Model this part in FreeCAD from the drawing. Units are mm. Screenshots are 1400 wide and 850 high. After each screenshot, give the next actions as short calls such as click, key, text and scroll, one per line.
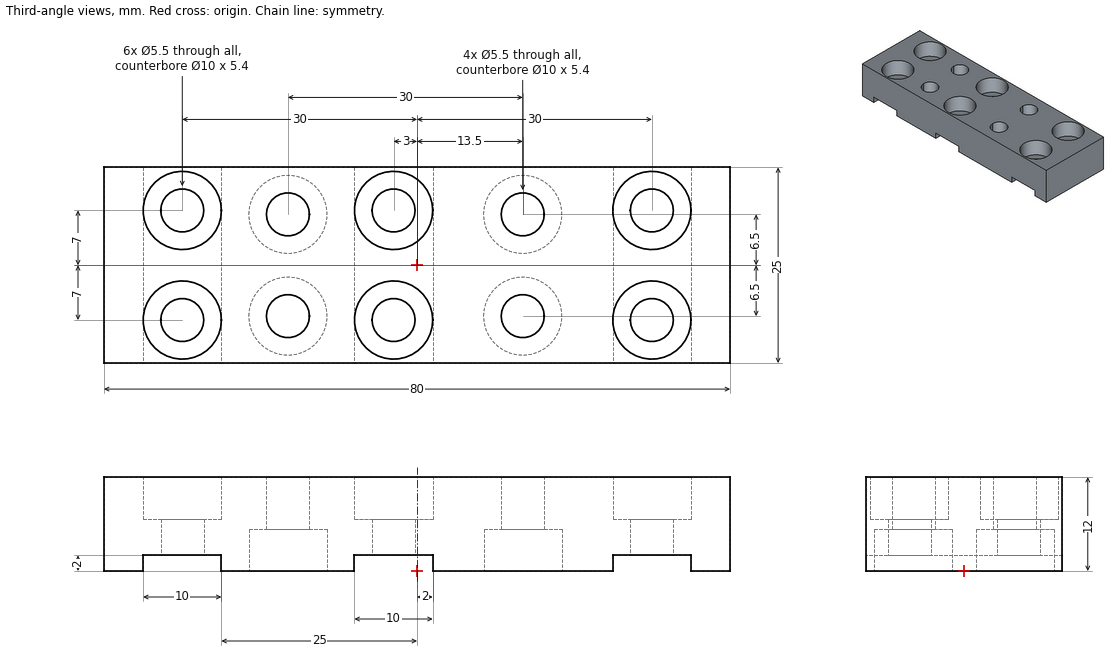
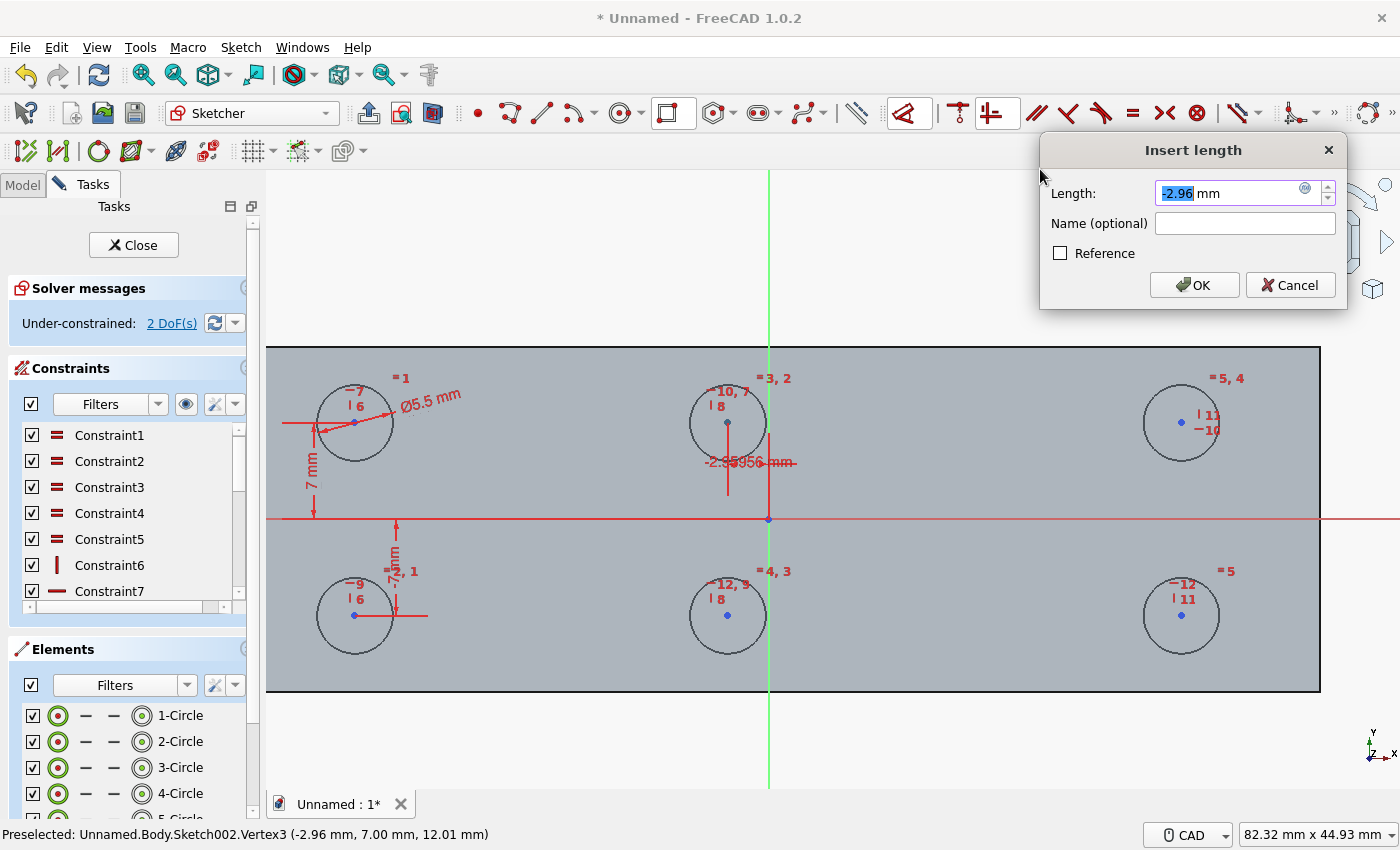
text(-3)
key(Return)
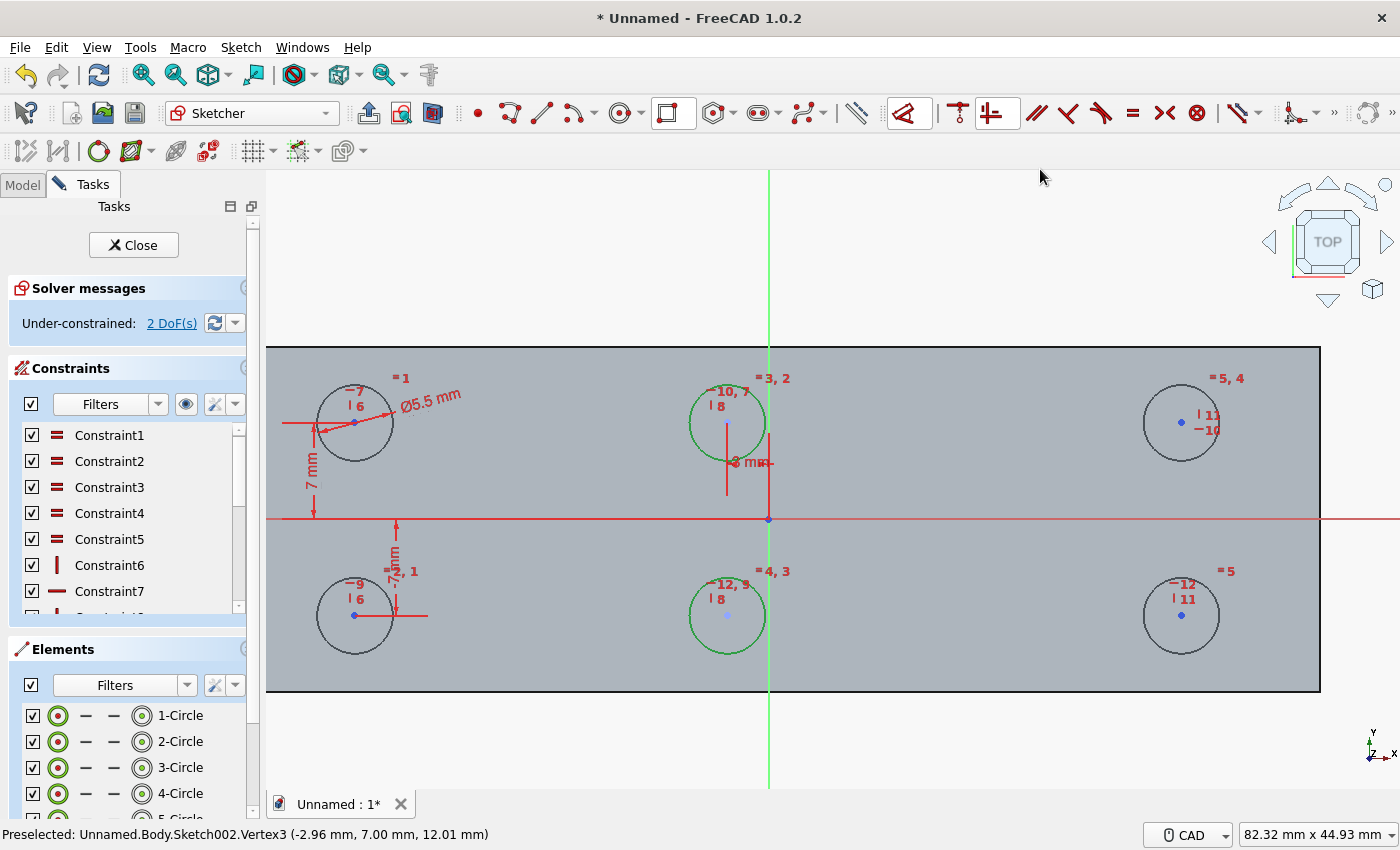
click(355, 423)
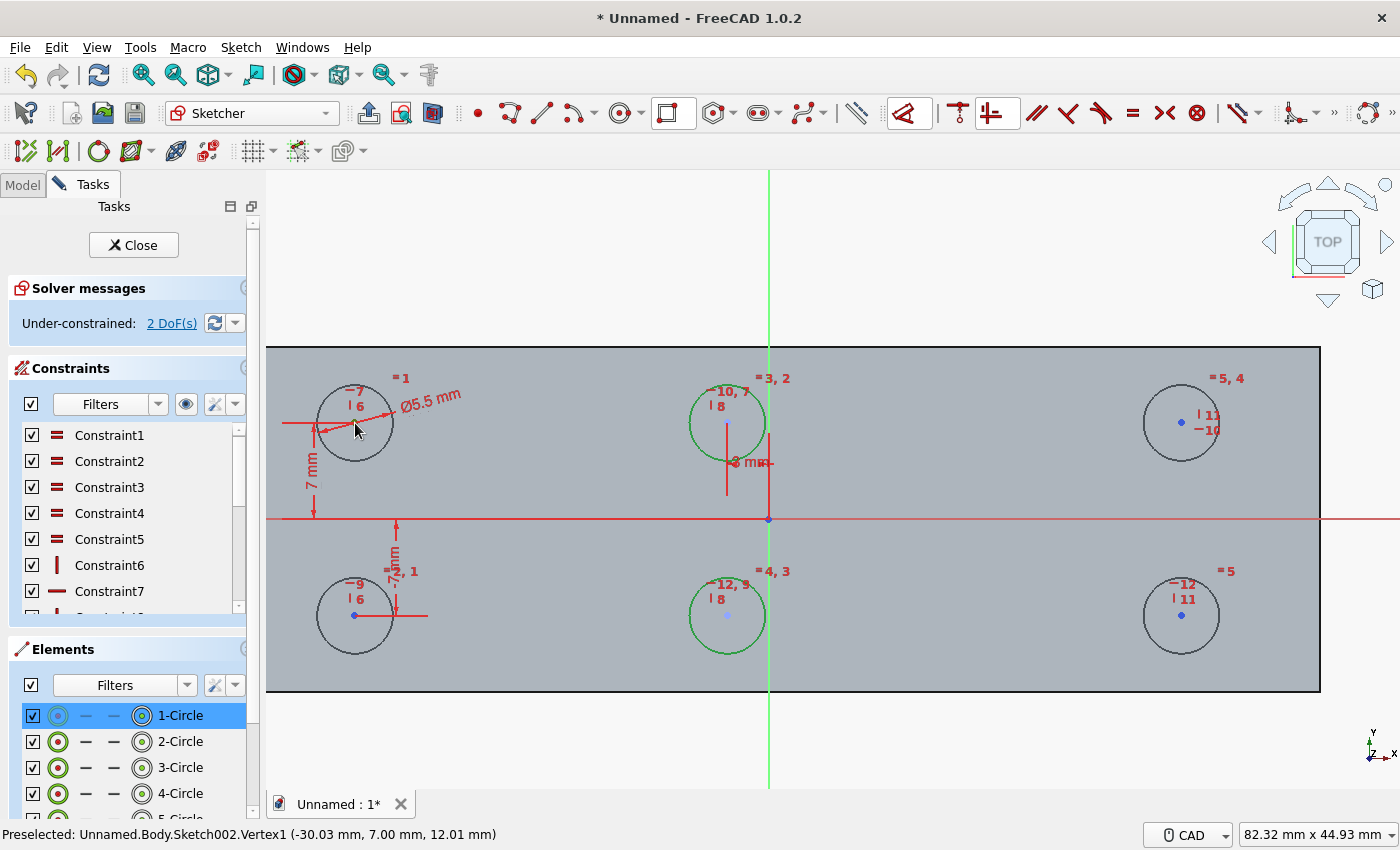
click(926, 114)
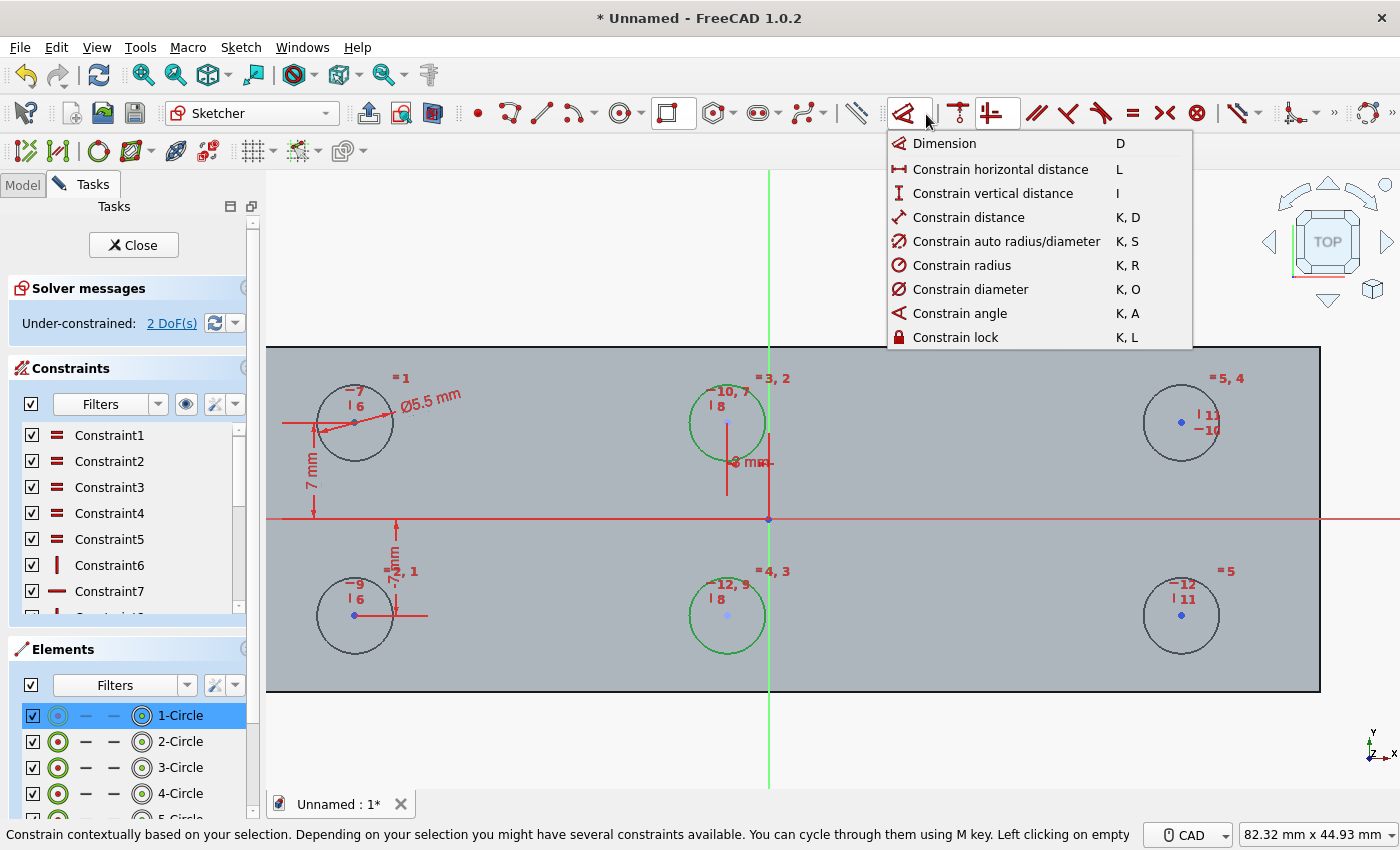
click(1040, 169)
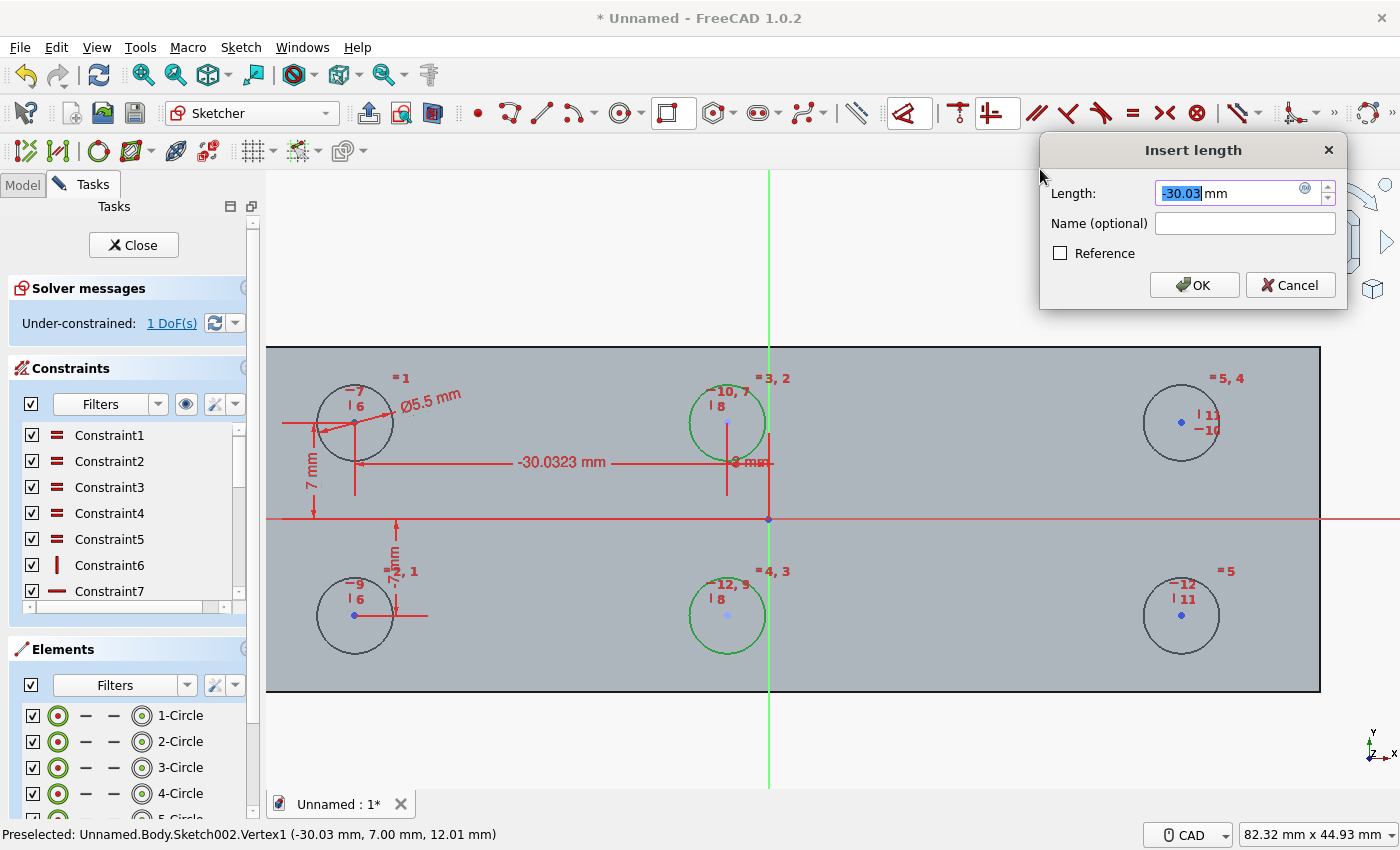
text(-30)
key(Return)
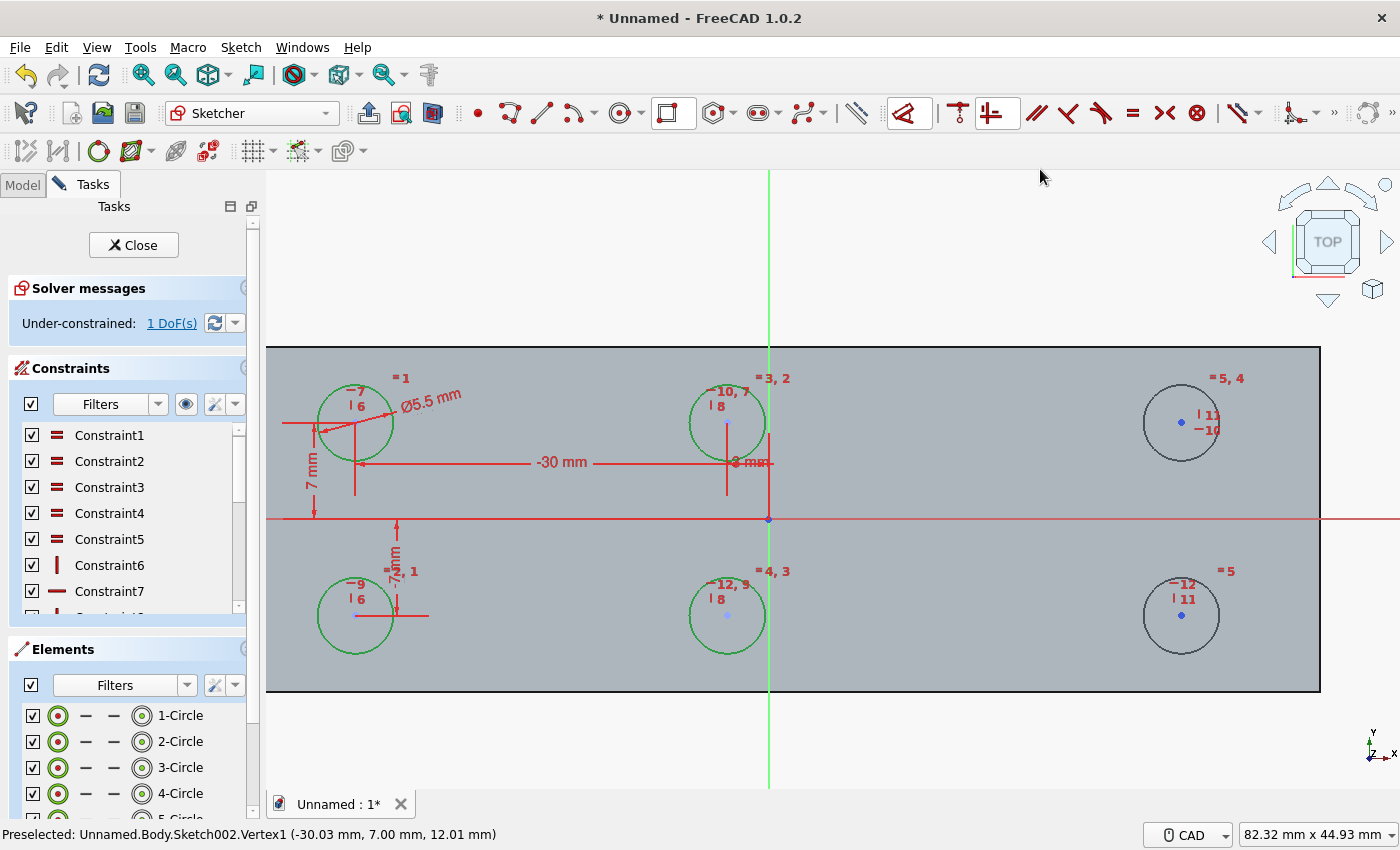
click(1181, 423)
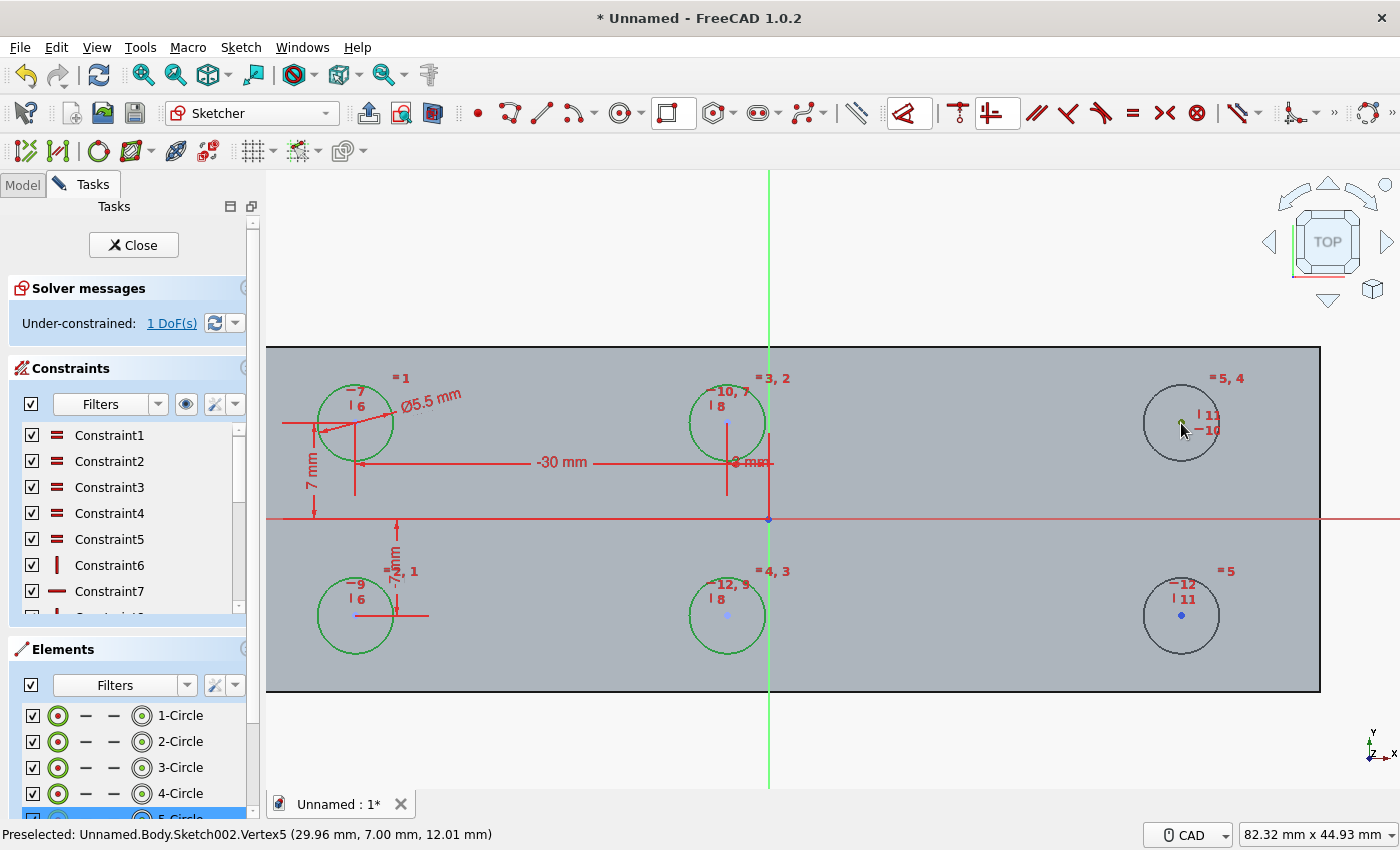
click(926, 114)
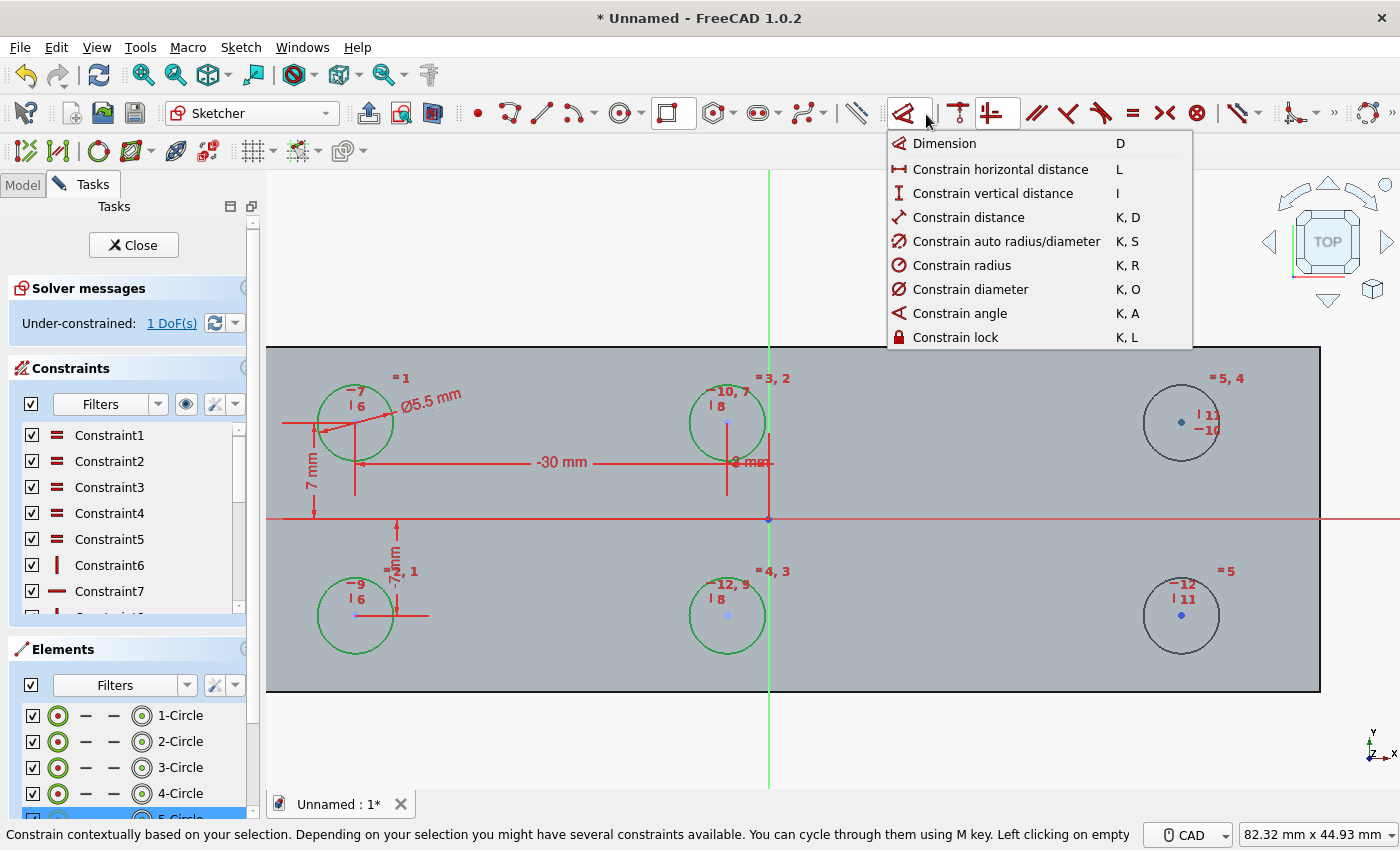
click(1040, 169)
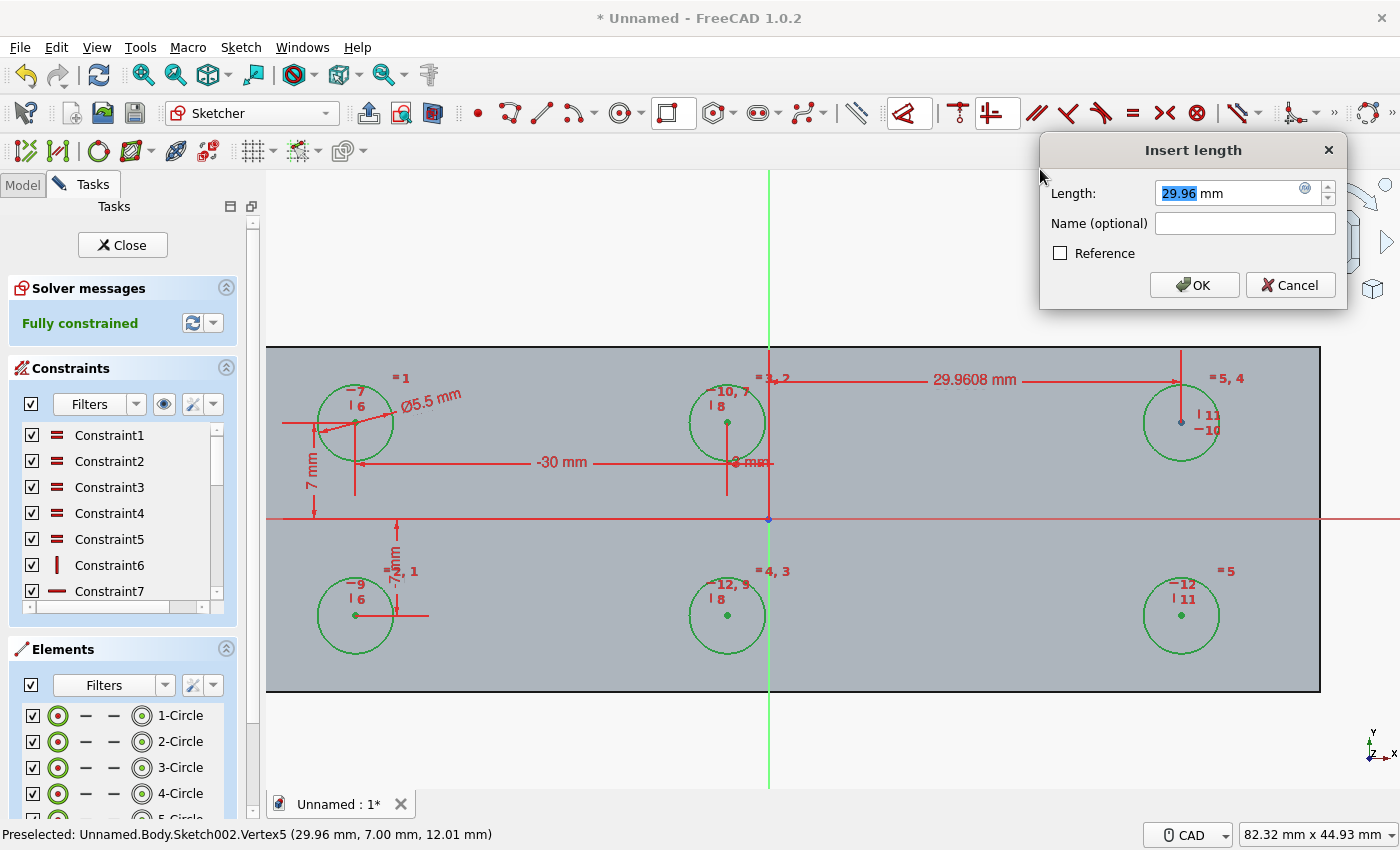
text(30)
key(Return)